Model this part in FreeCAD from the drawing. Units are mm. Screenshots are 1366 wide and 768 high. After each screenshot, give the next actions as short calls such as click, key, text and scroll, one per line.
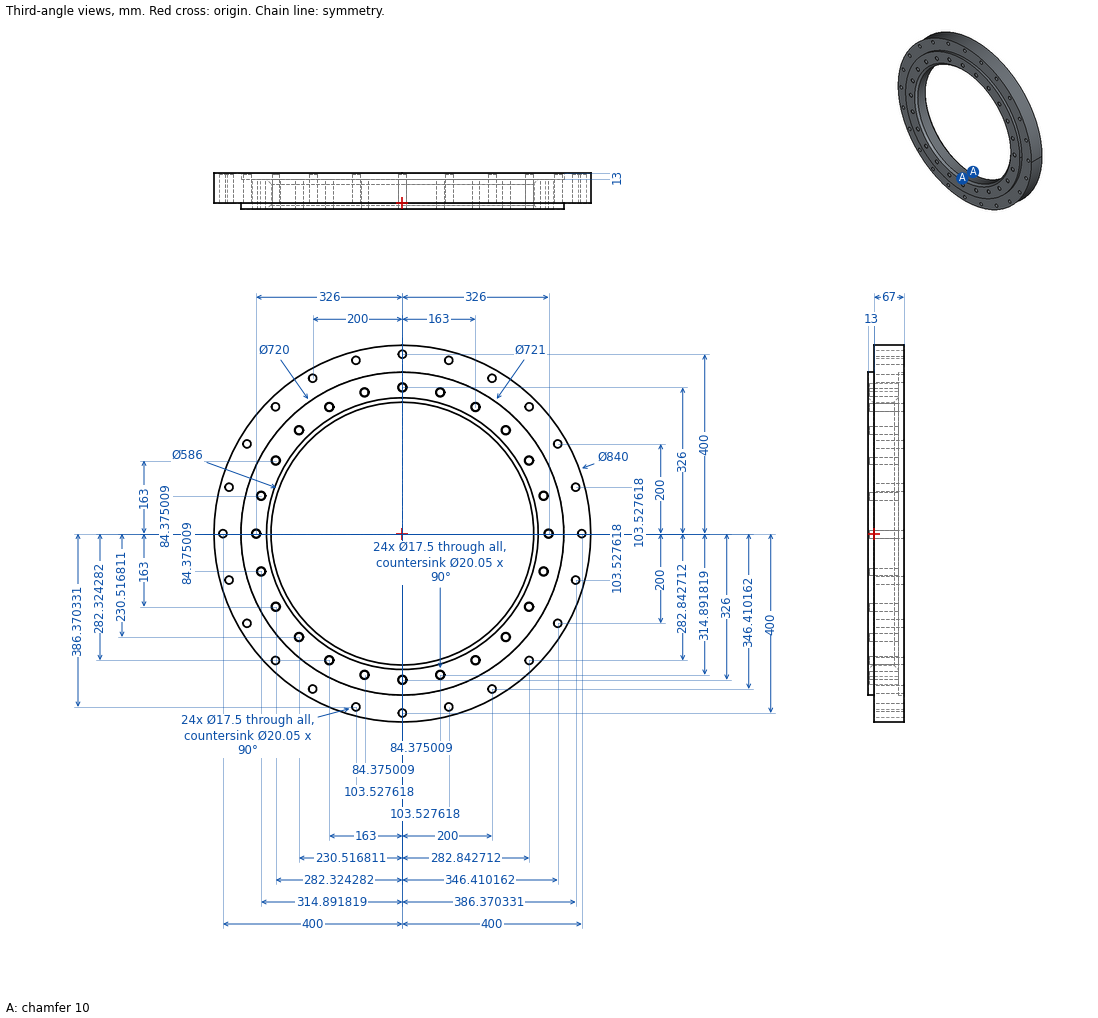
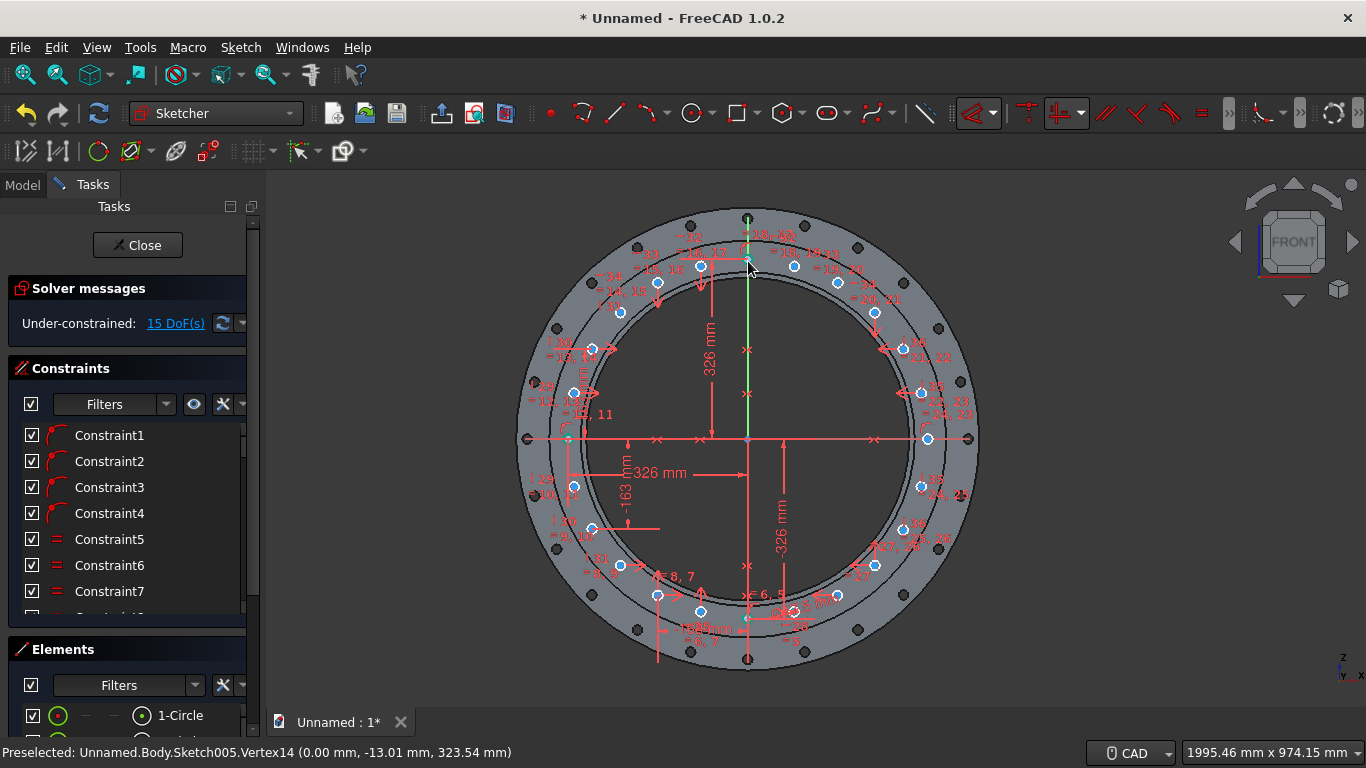
click(838, 283)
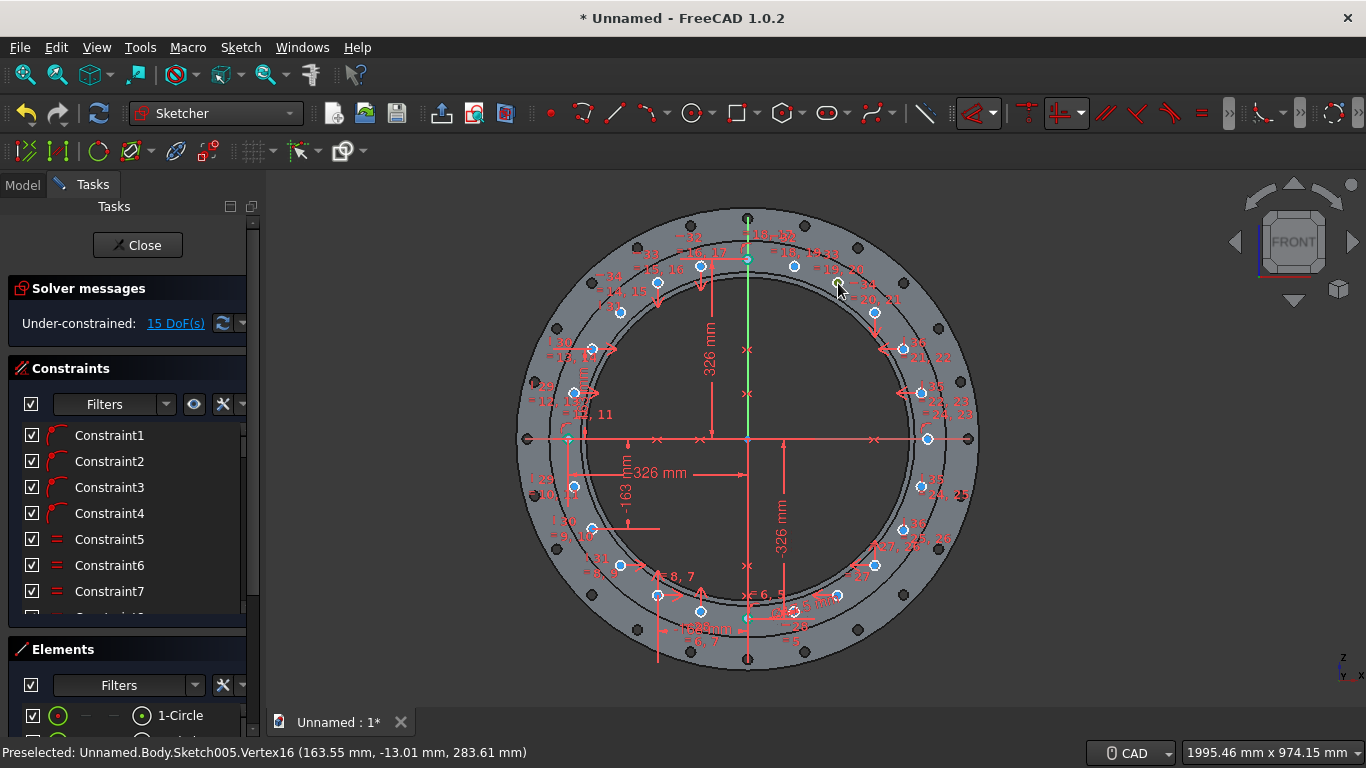
key(l)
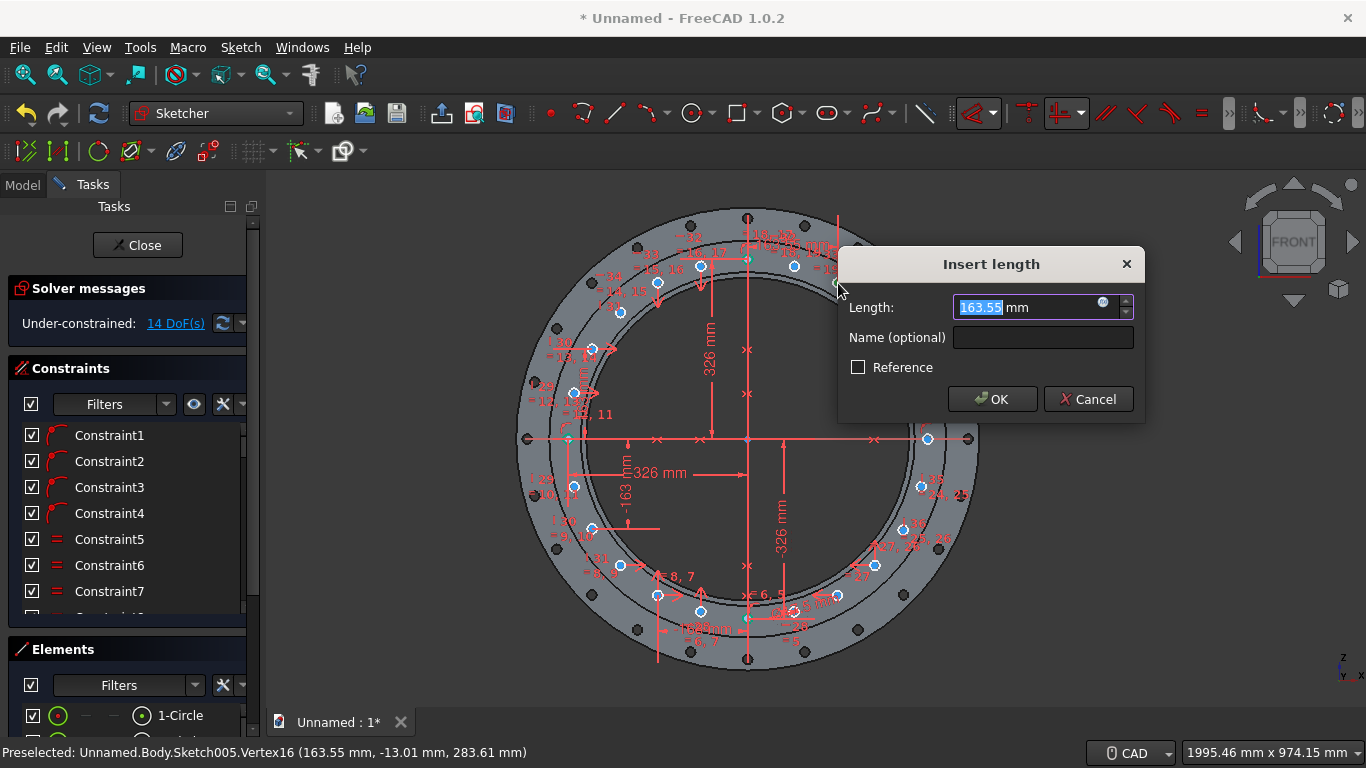
text(163)
key(Return)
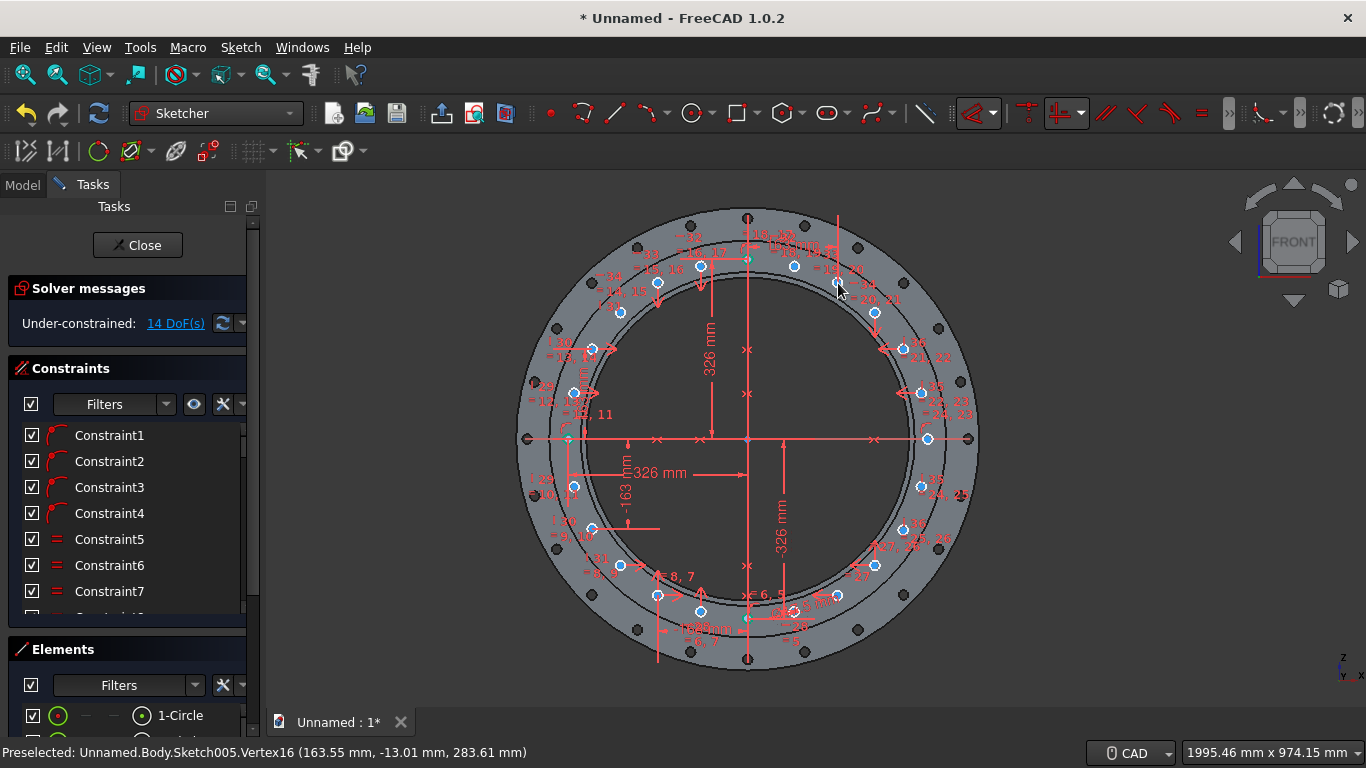
click(928, 439)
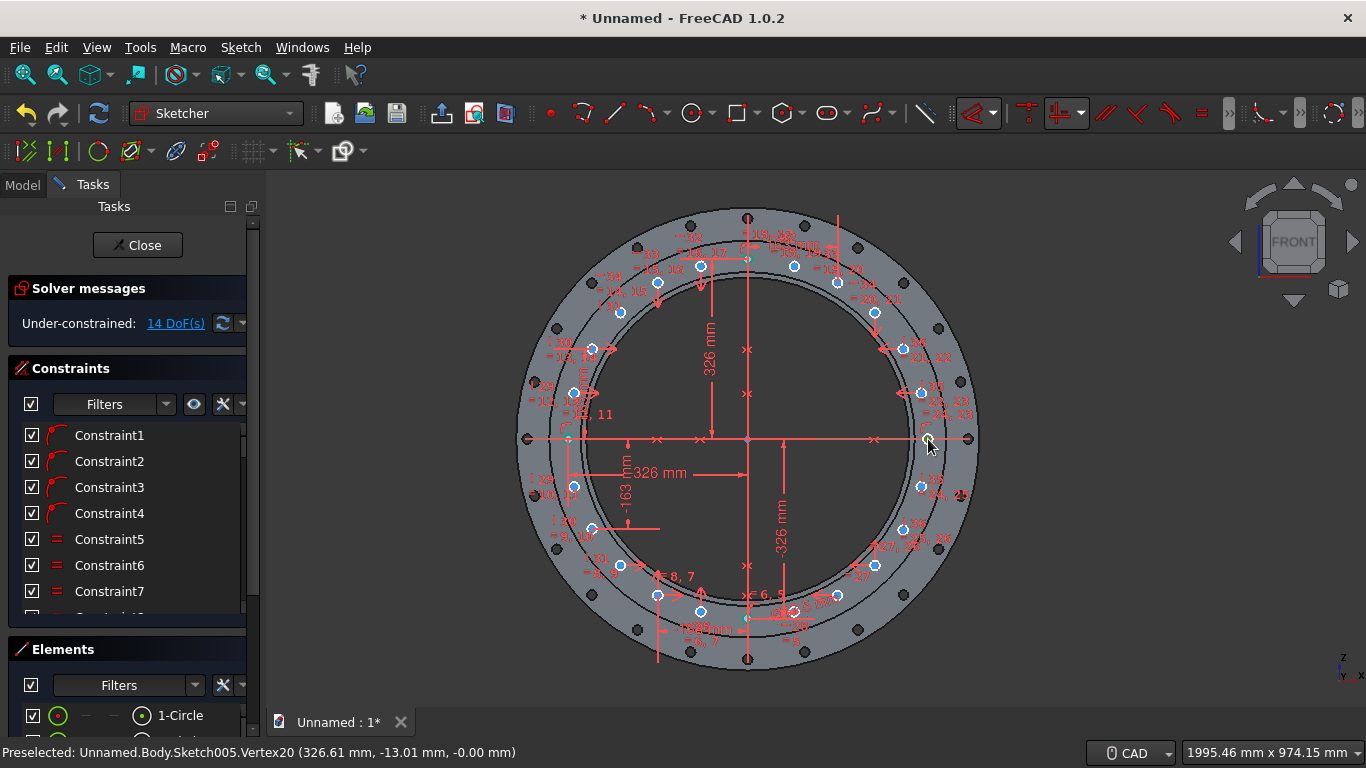
key(l)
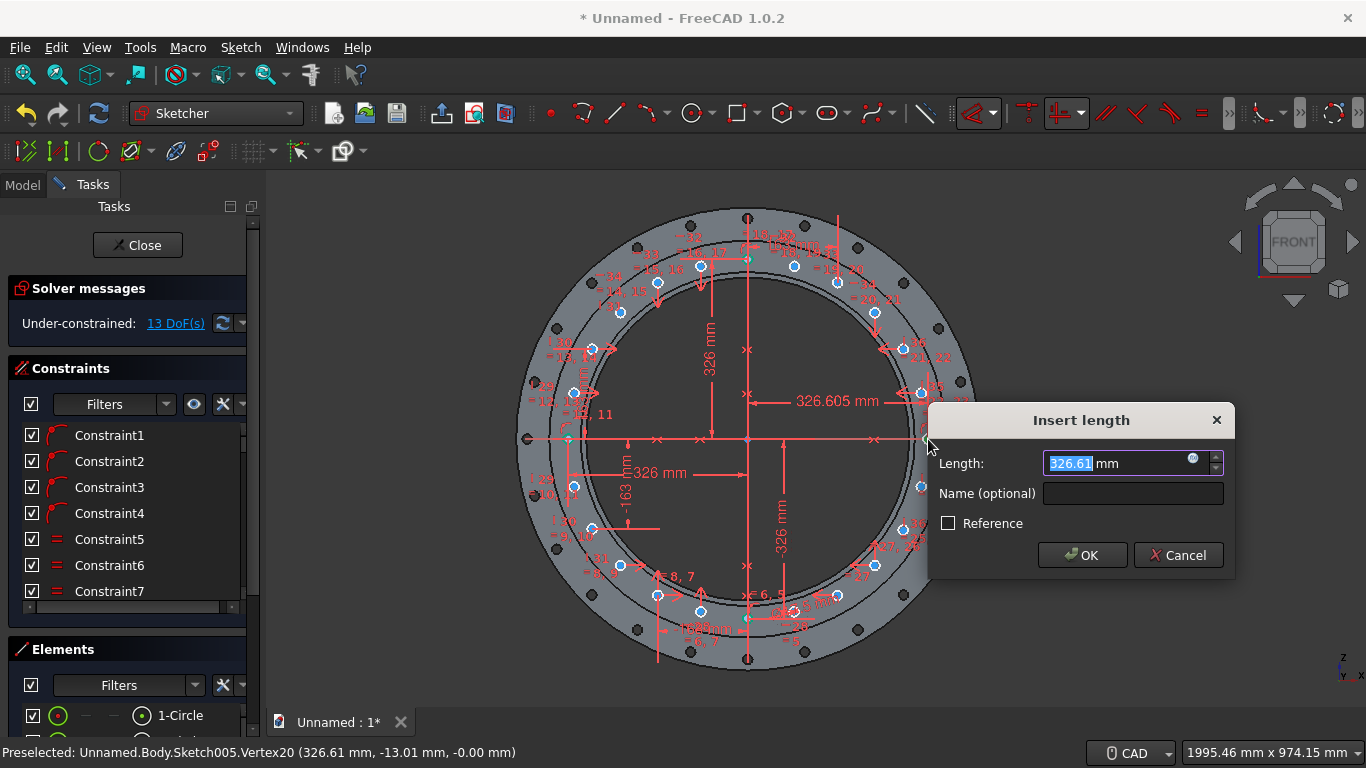
text(326)
key(Return)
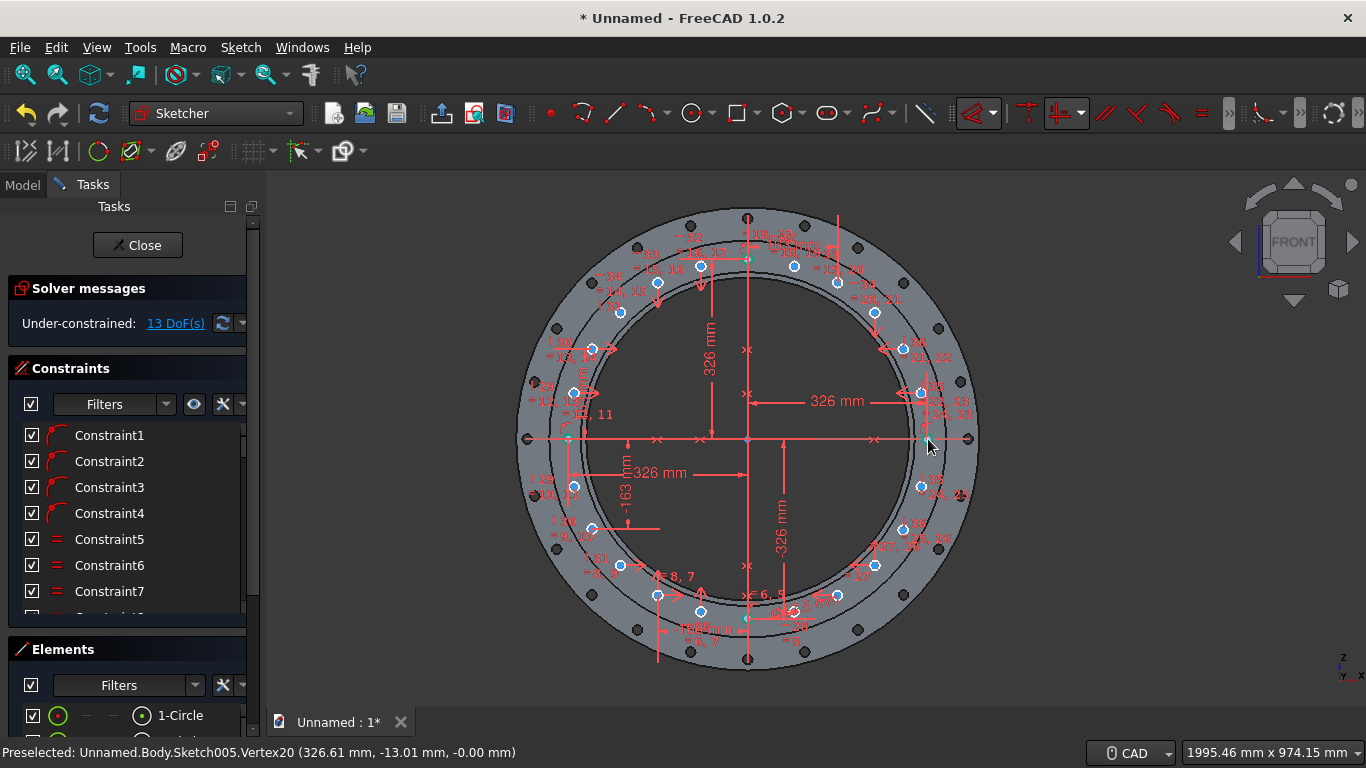
scroll(903, 530, up, 4)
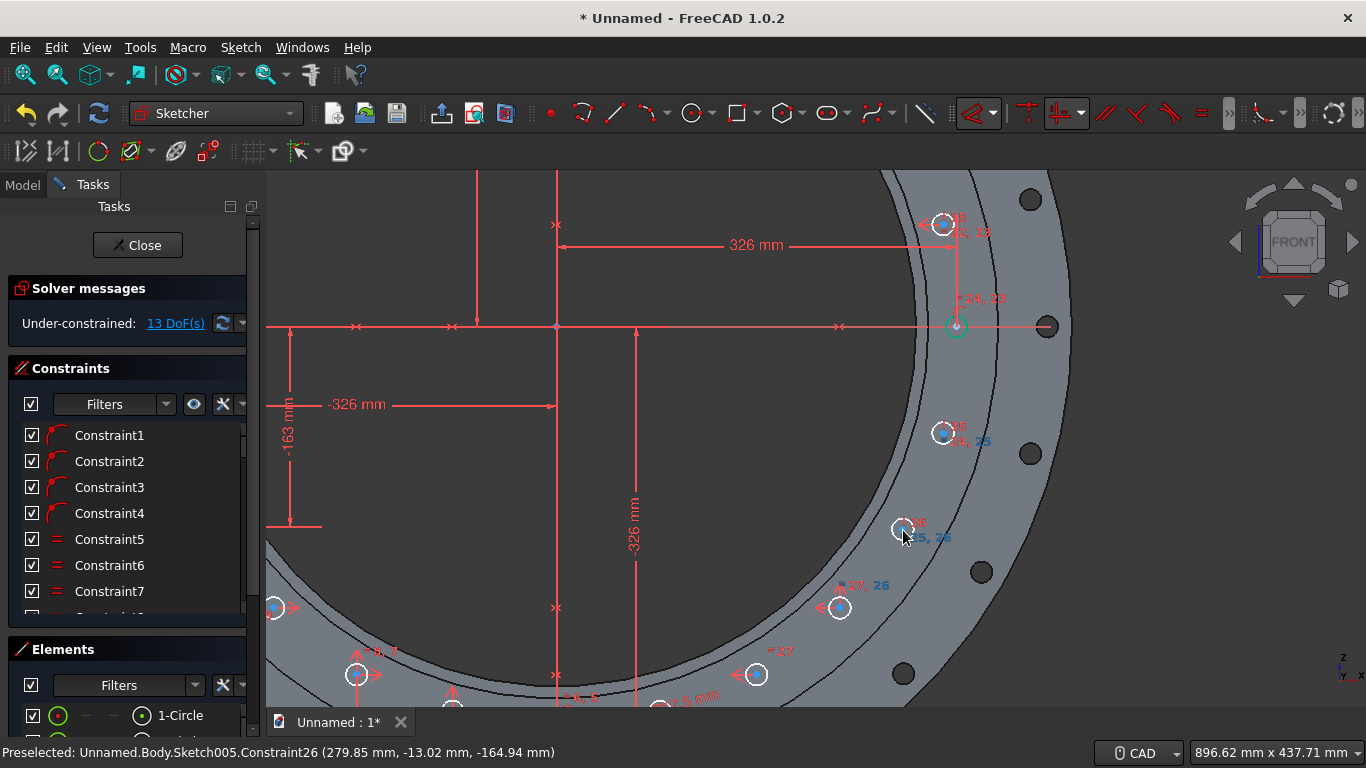
scroll(903, 529, up, 4)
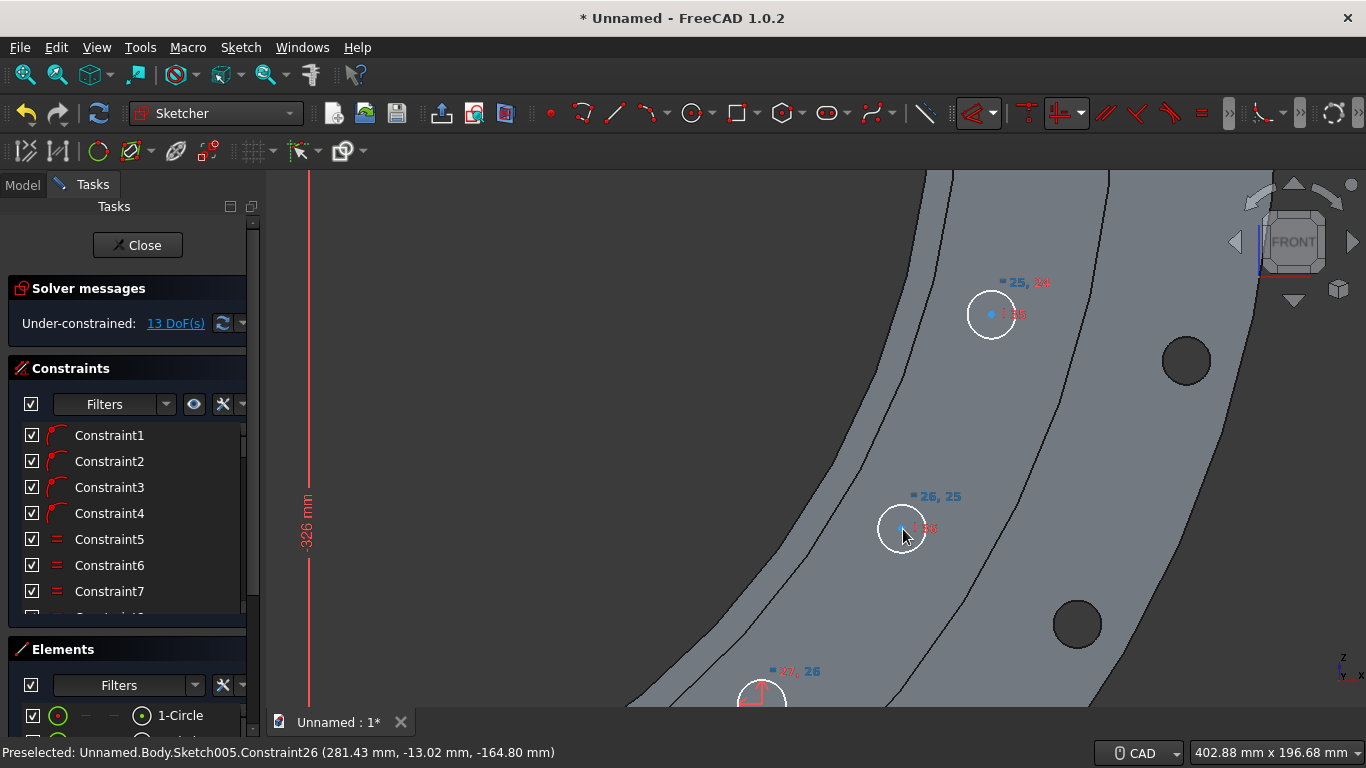
click(902, 529)